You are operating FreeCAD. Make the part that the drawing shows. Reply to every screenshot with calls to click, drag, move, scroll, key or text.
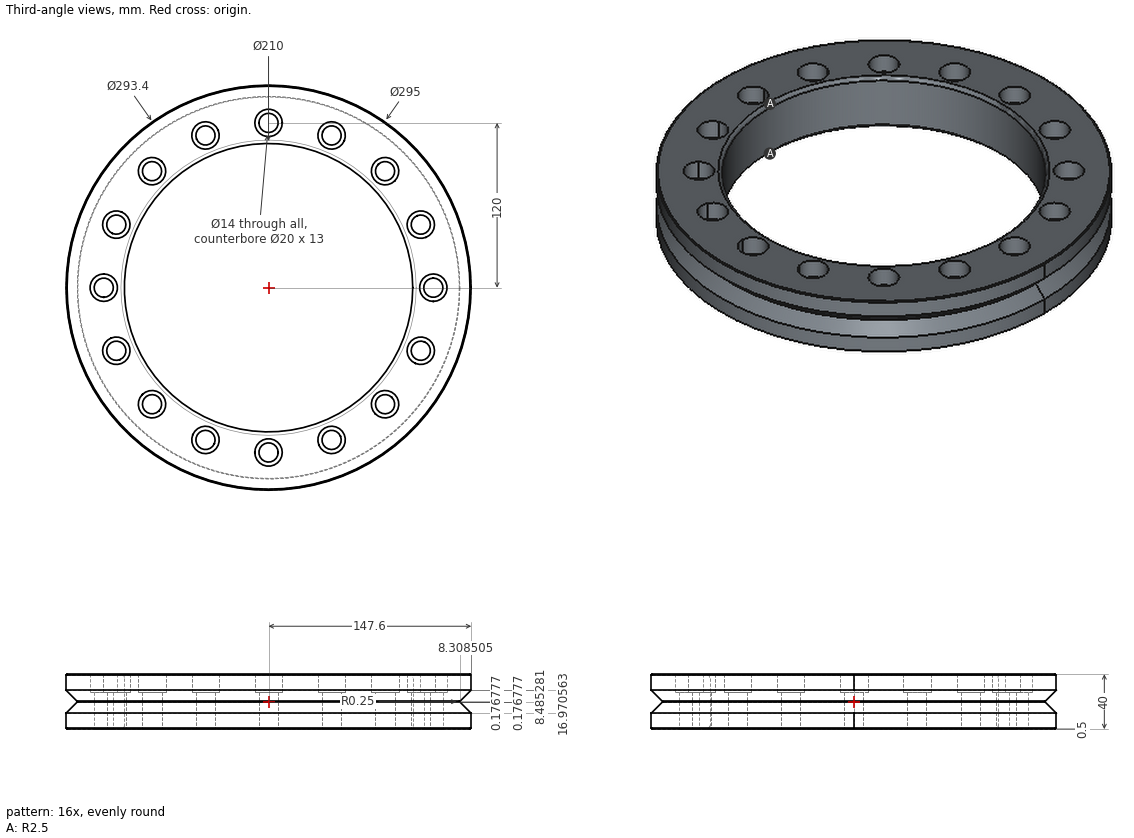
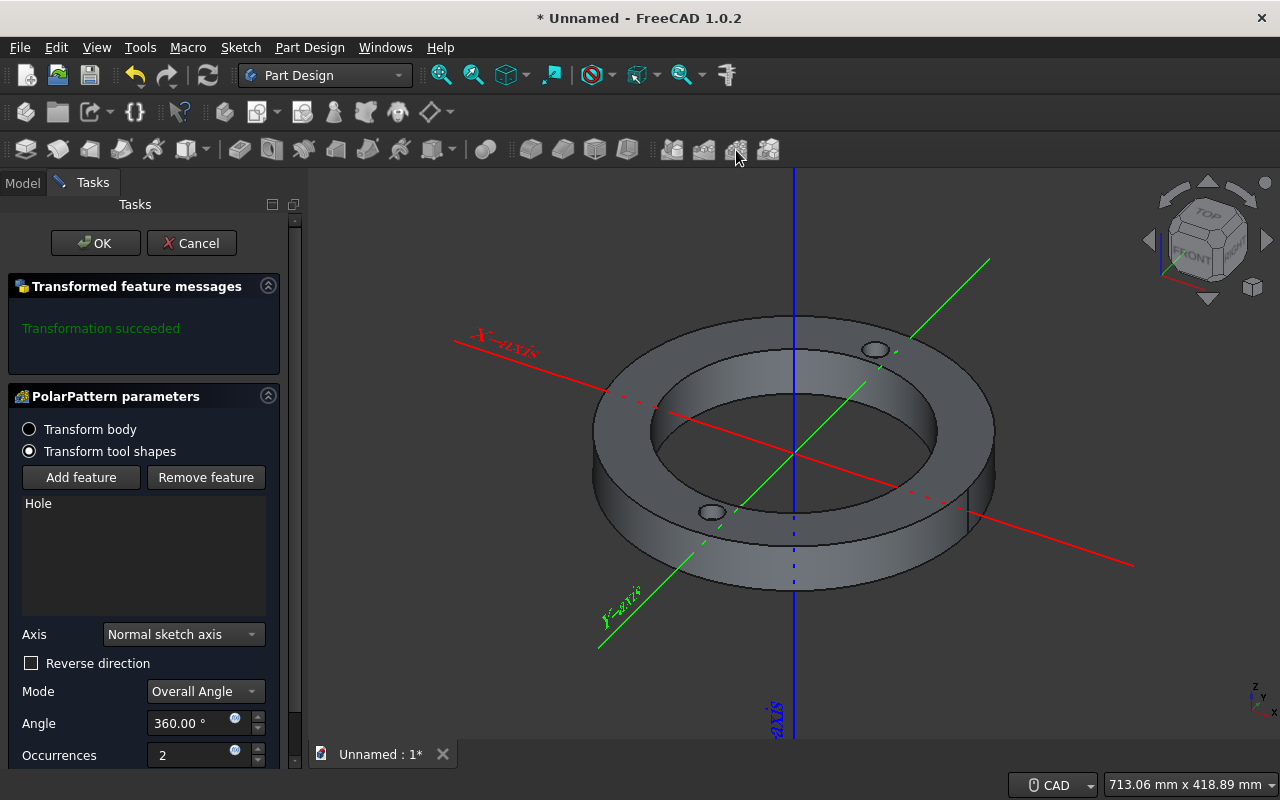
click(184, 634)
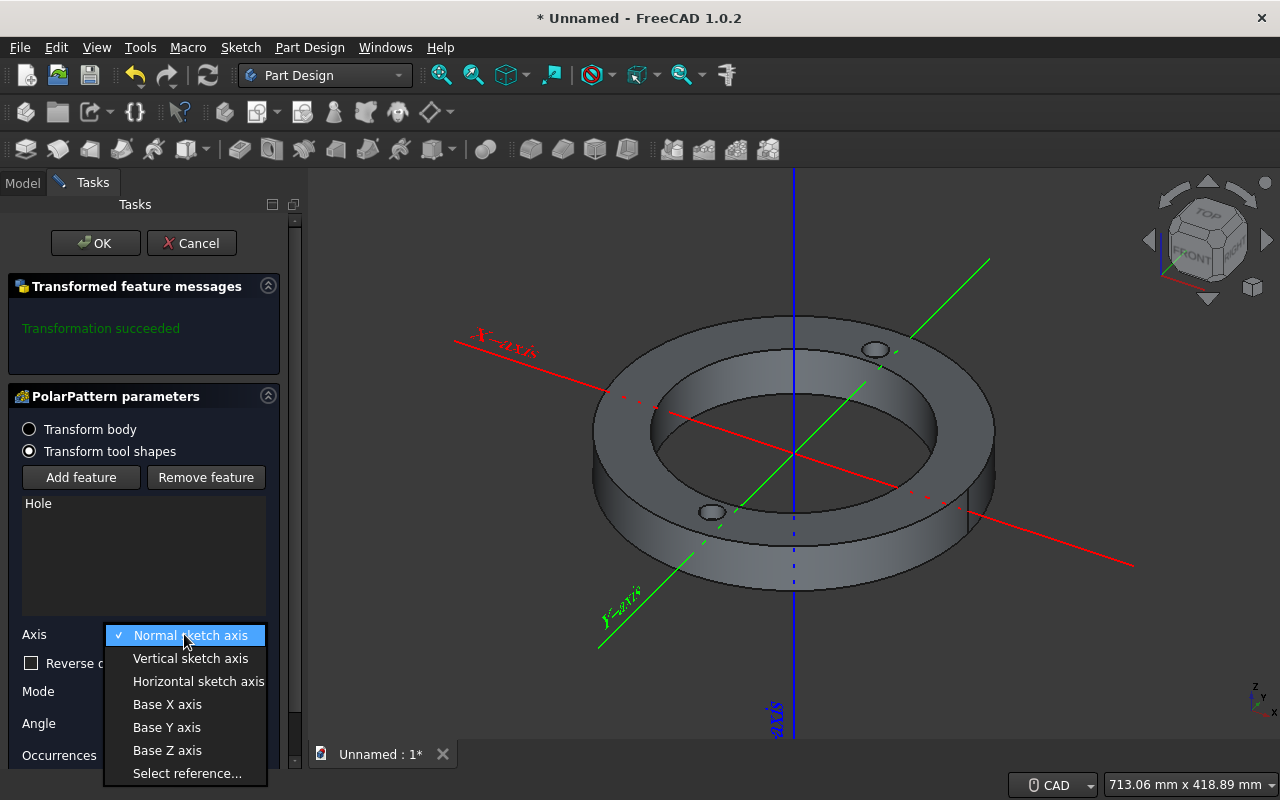
click(184, 750)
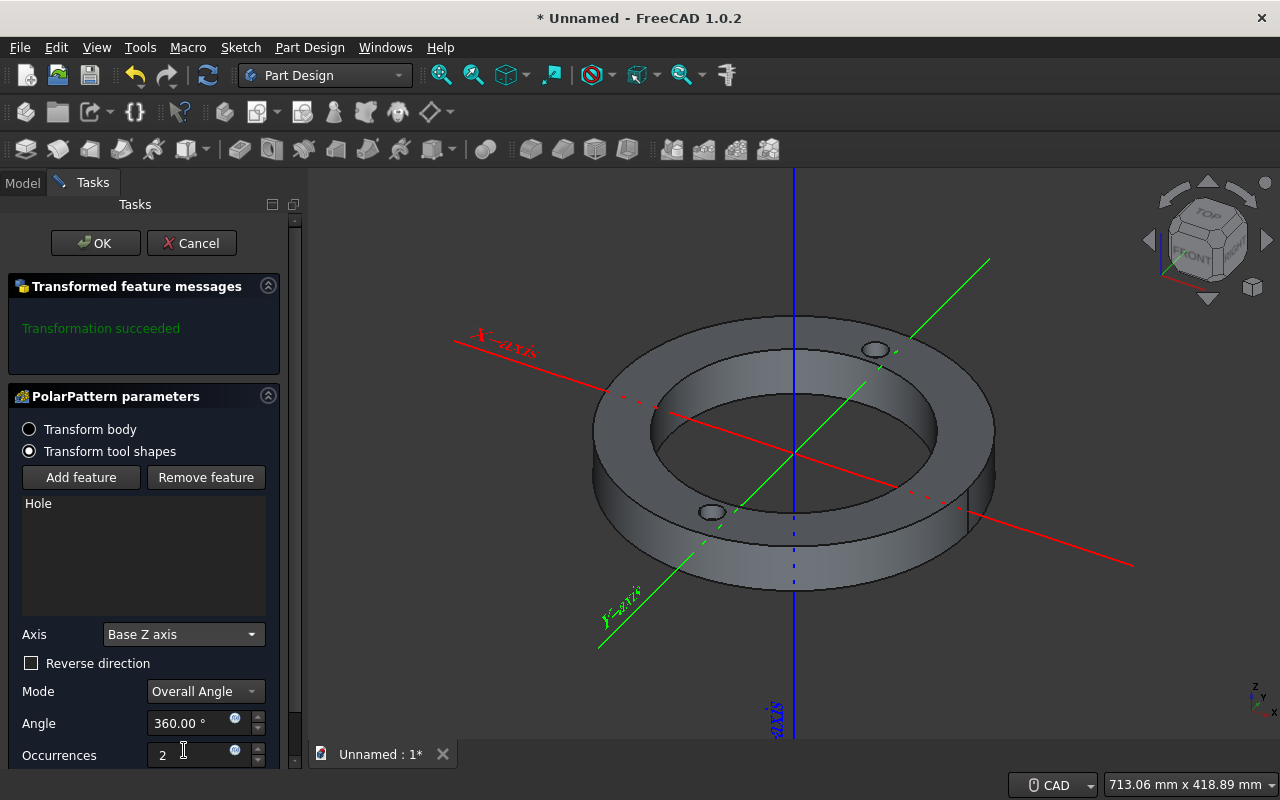
triple_click(198, 755)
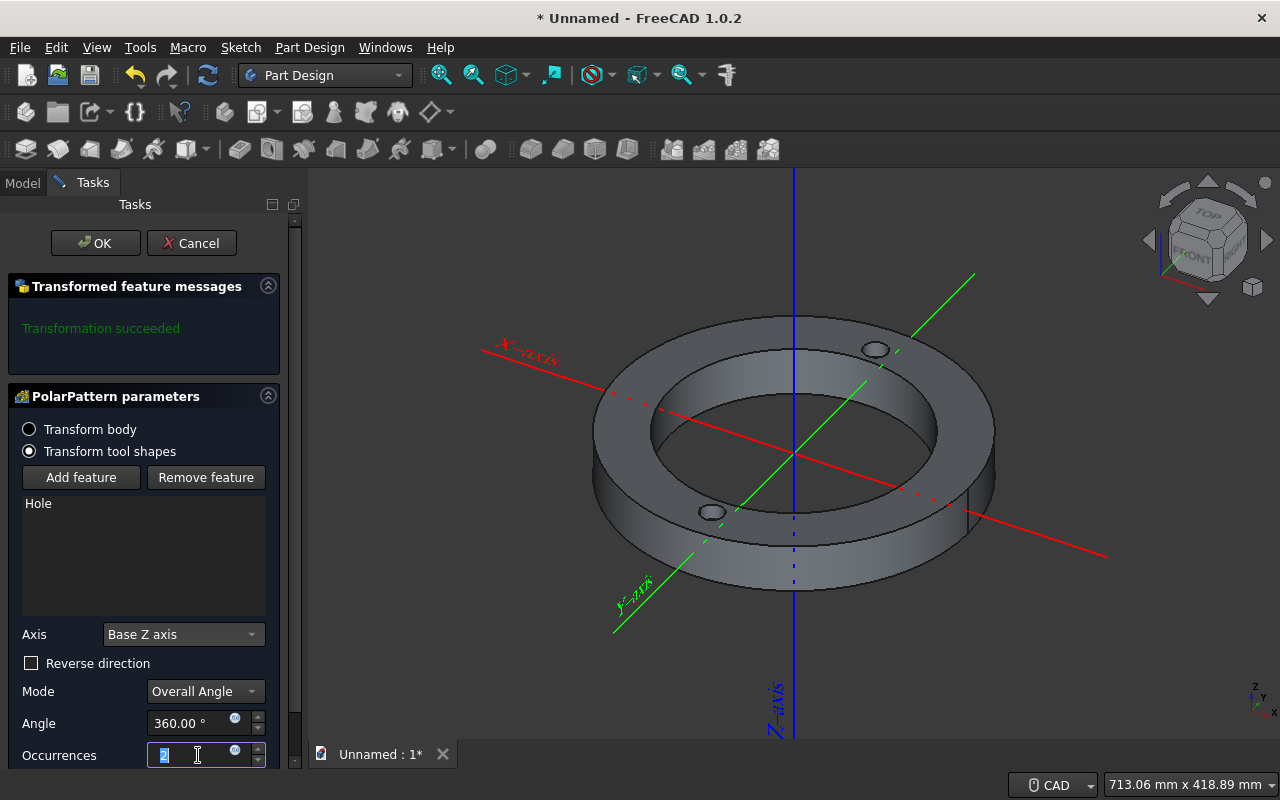
text(16)
key(Tab)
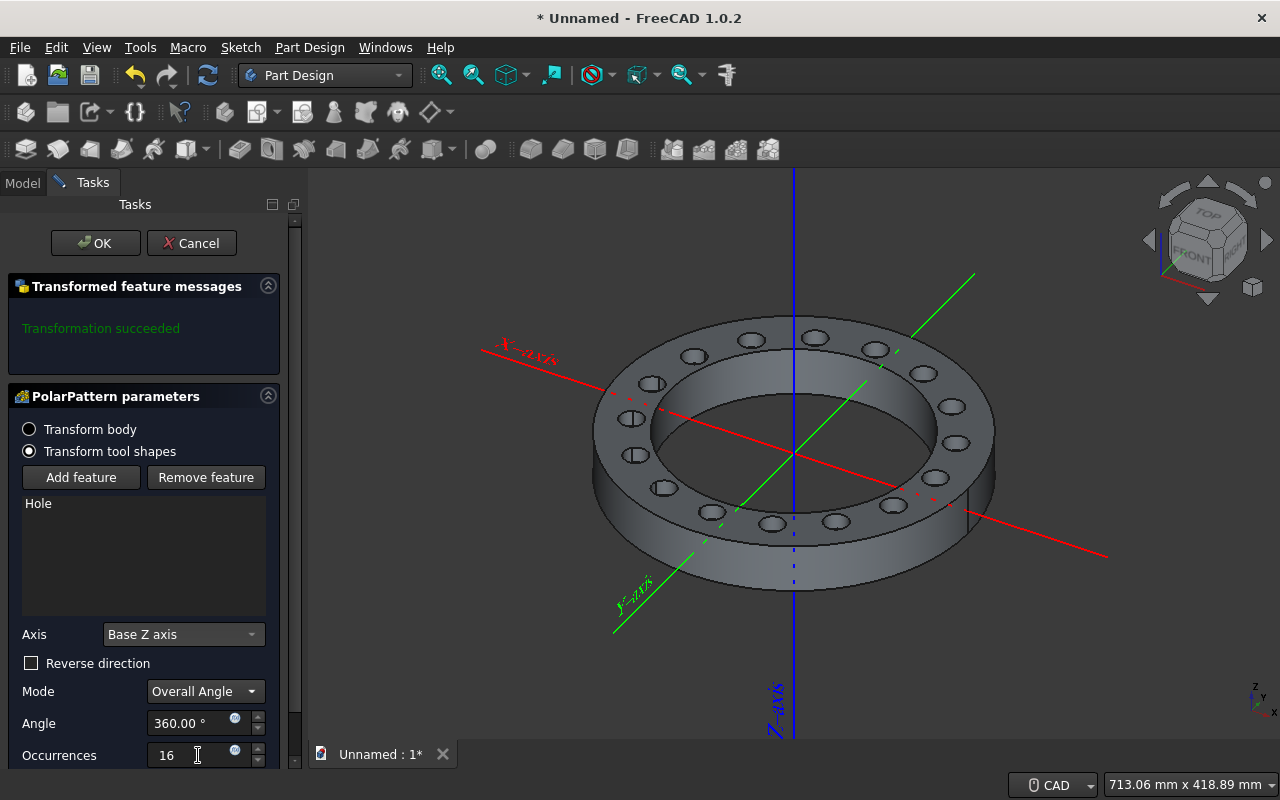
click(96, 243)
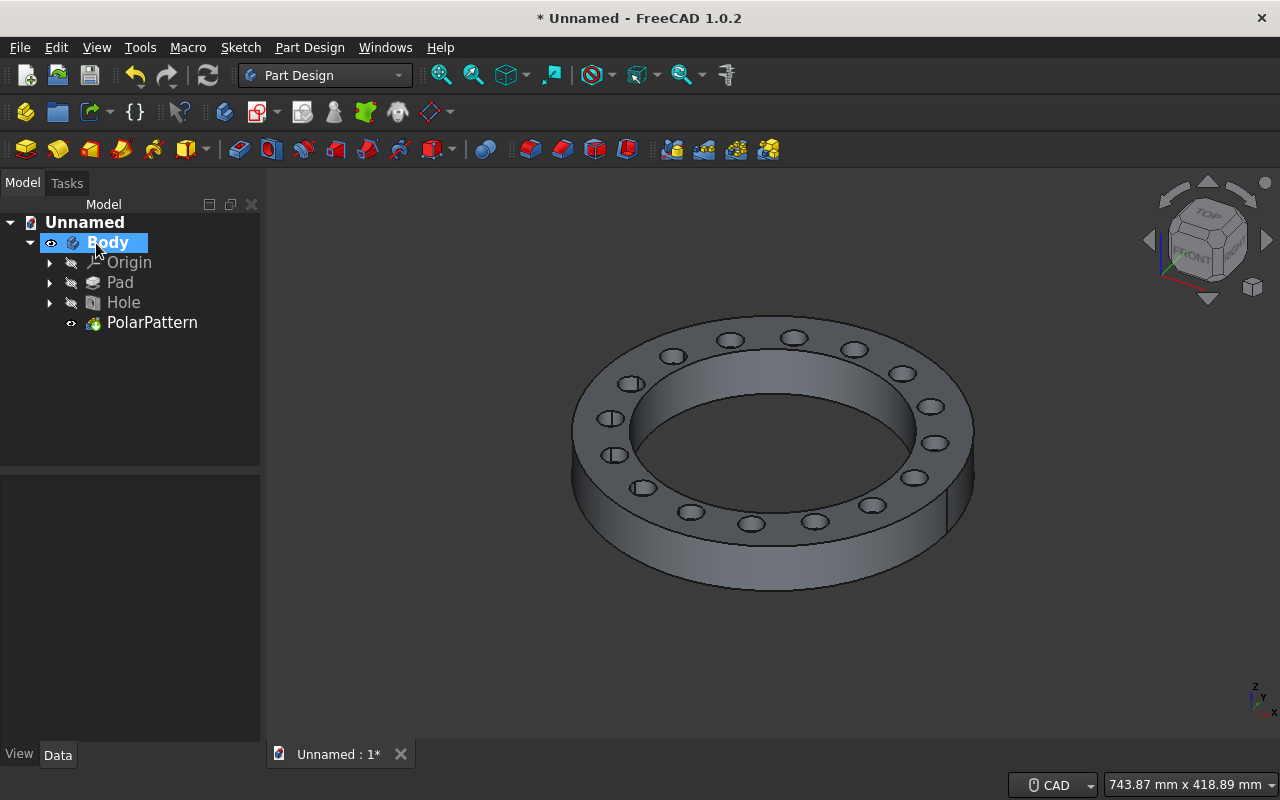
click(258, 112)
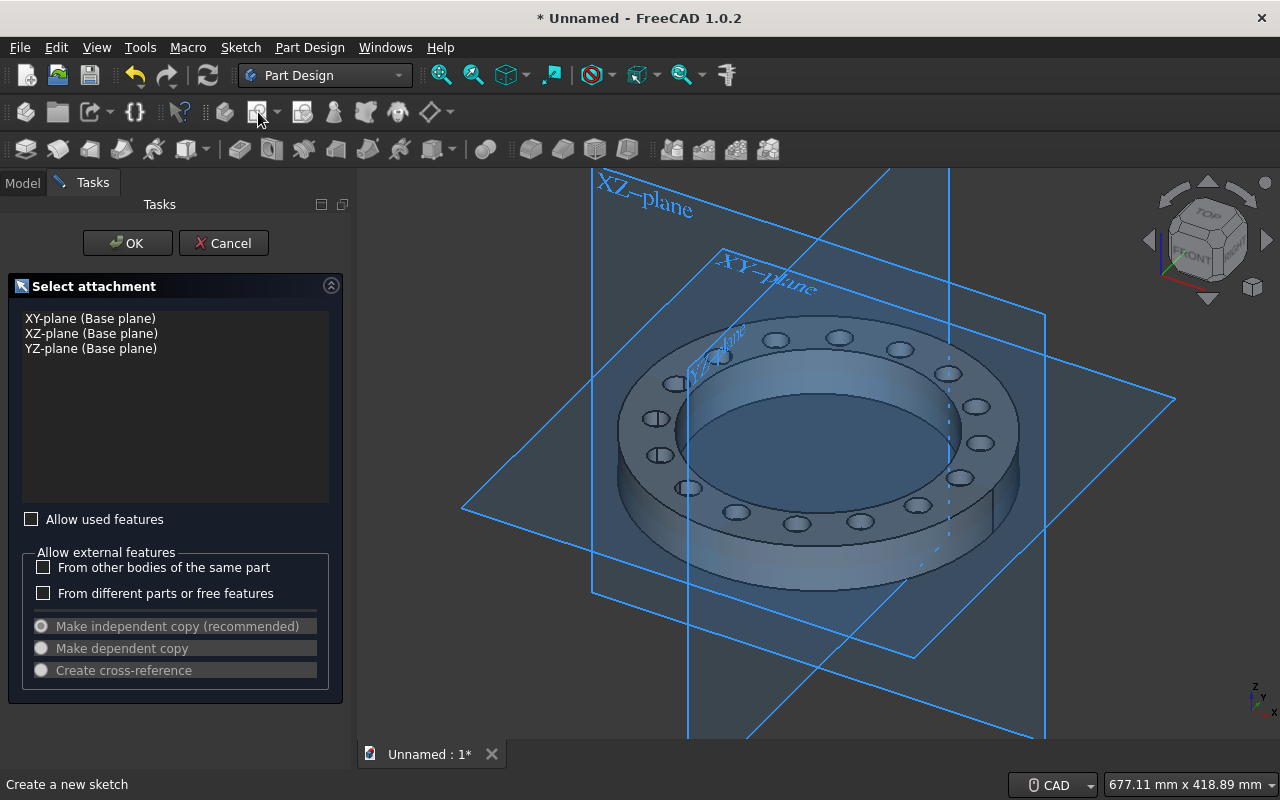
click(82, 334)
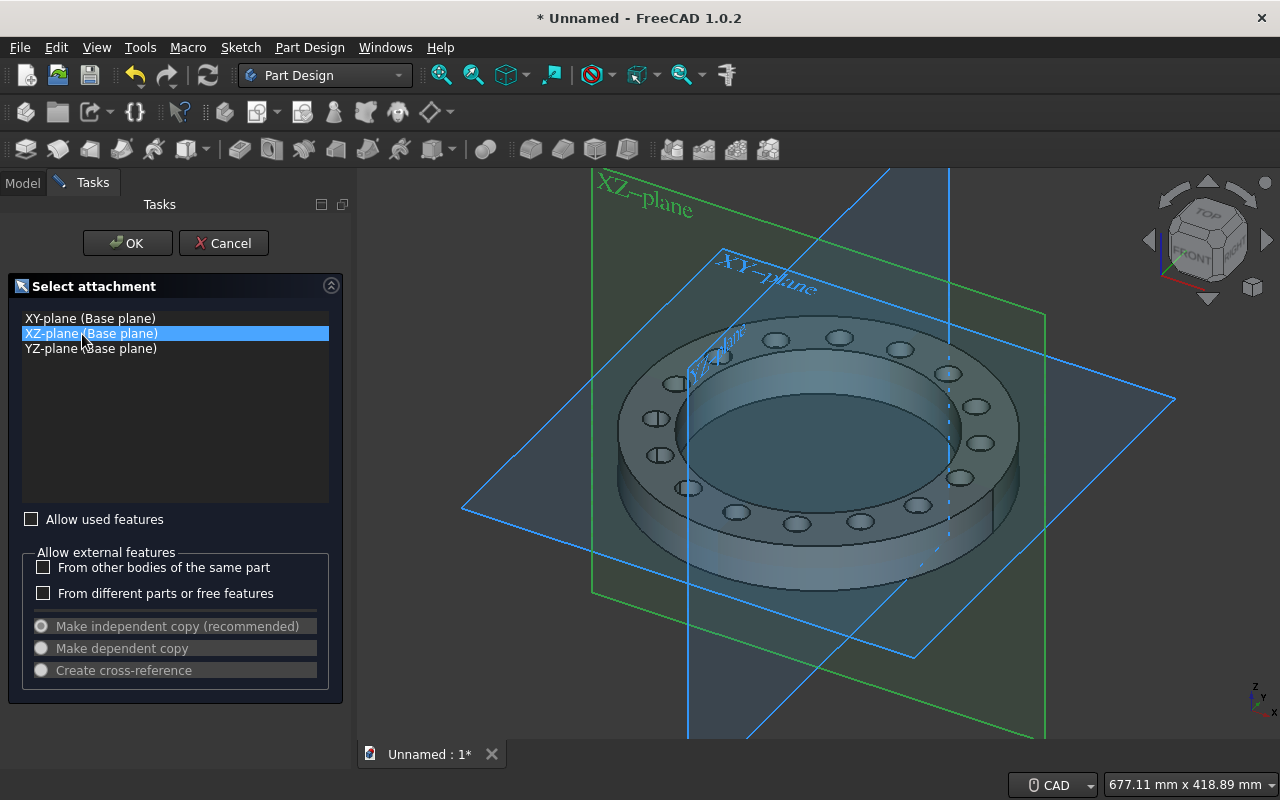
click(128, 243)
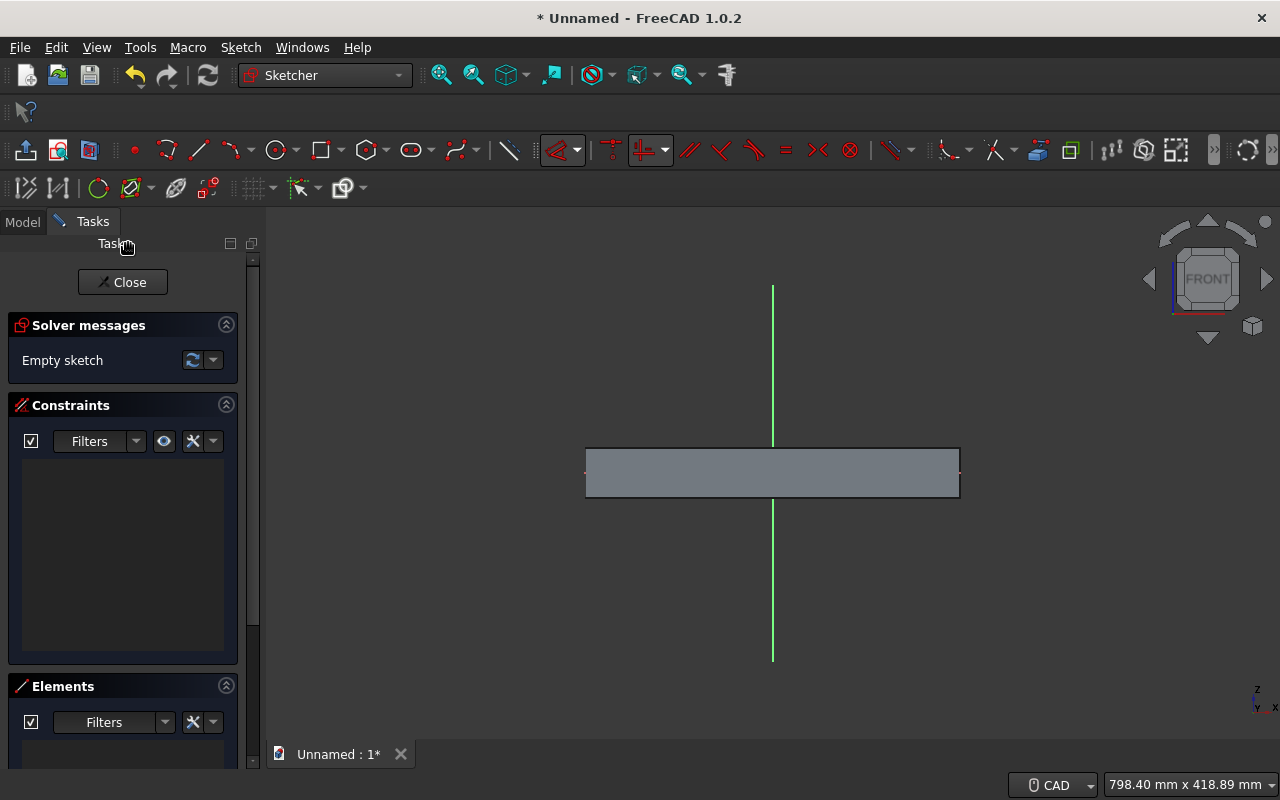
key(q)
key(s)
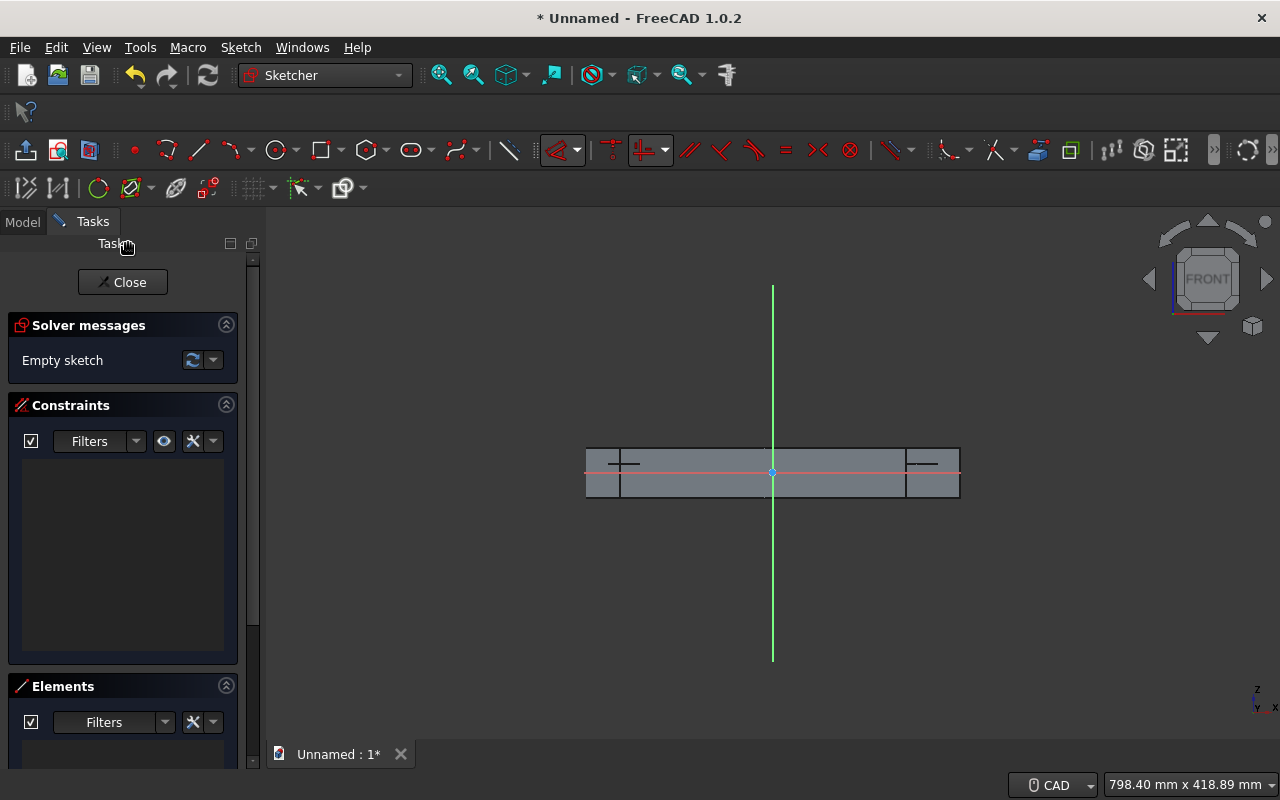
scroll(971, 473, up, 14)